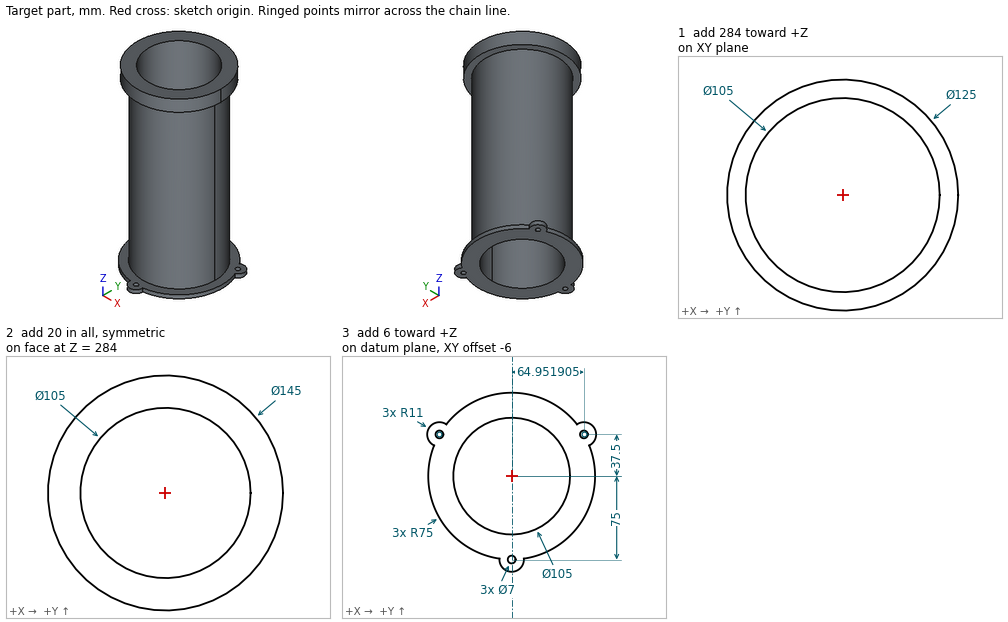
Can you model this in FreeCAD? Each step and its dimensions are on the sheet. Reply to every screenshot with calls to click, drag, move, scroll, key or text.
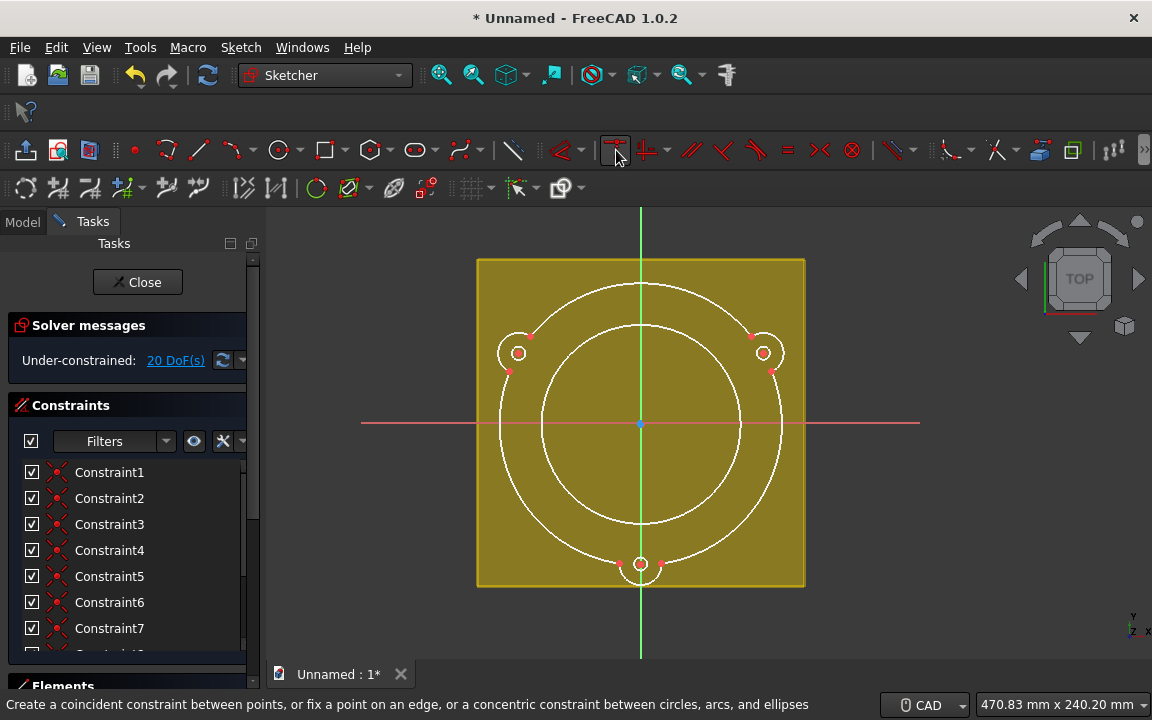
click(711, 354)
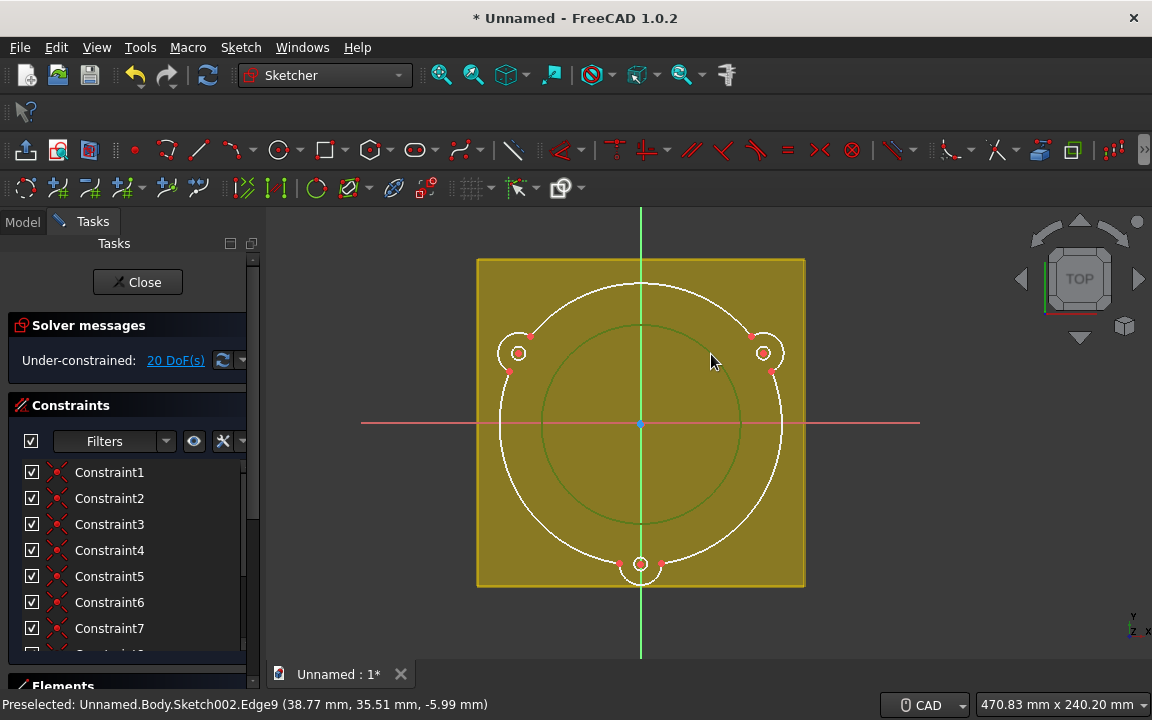
click(501, 447)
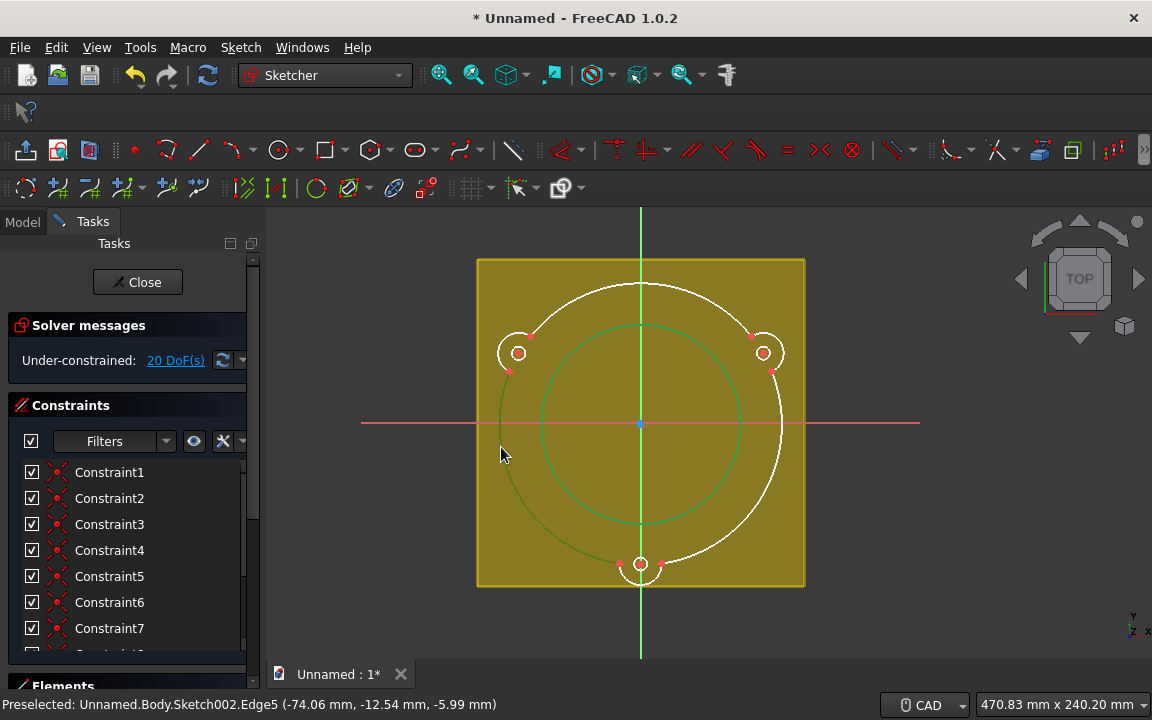
click(616, 150)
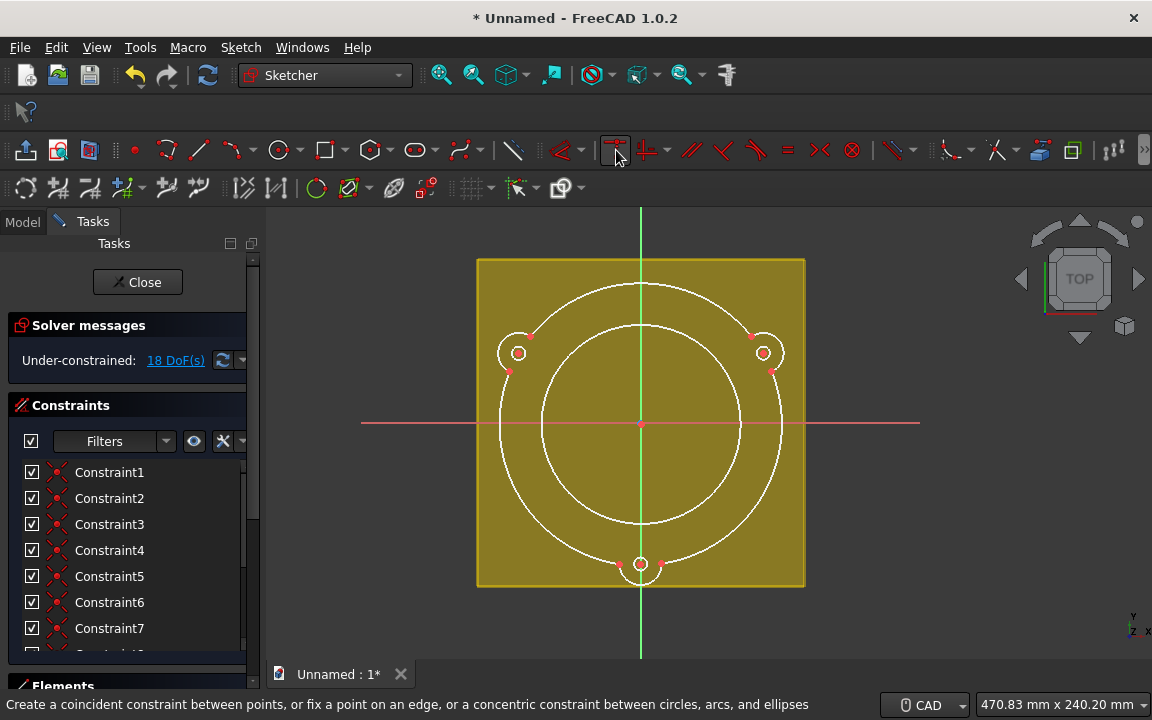
scroll(641, 424, up, 10)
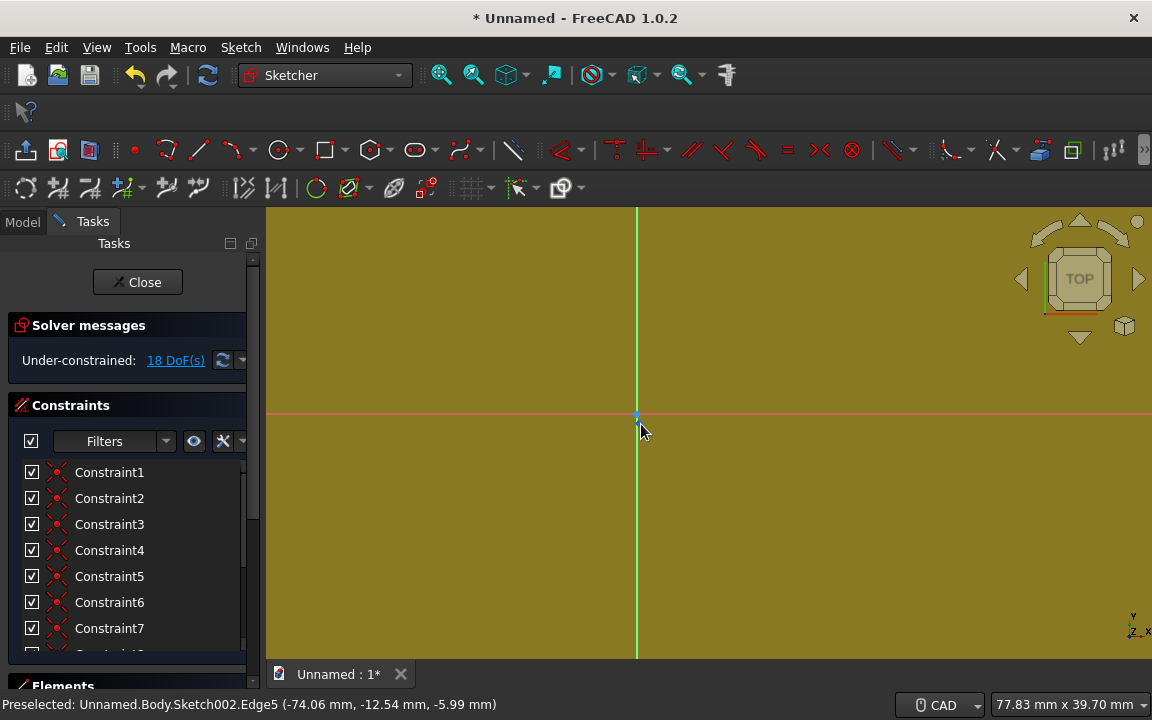
drag(627, 404, 649, 434)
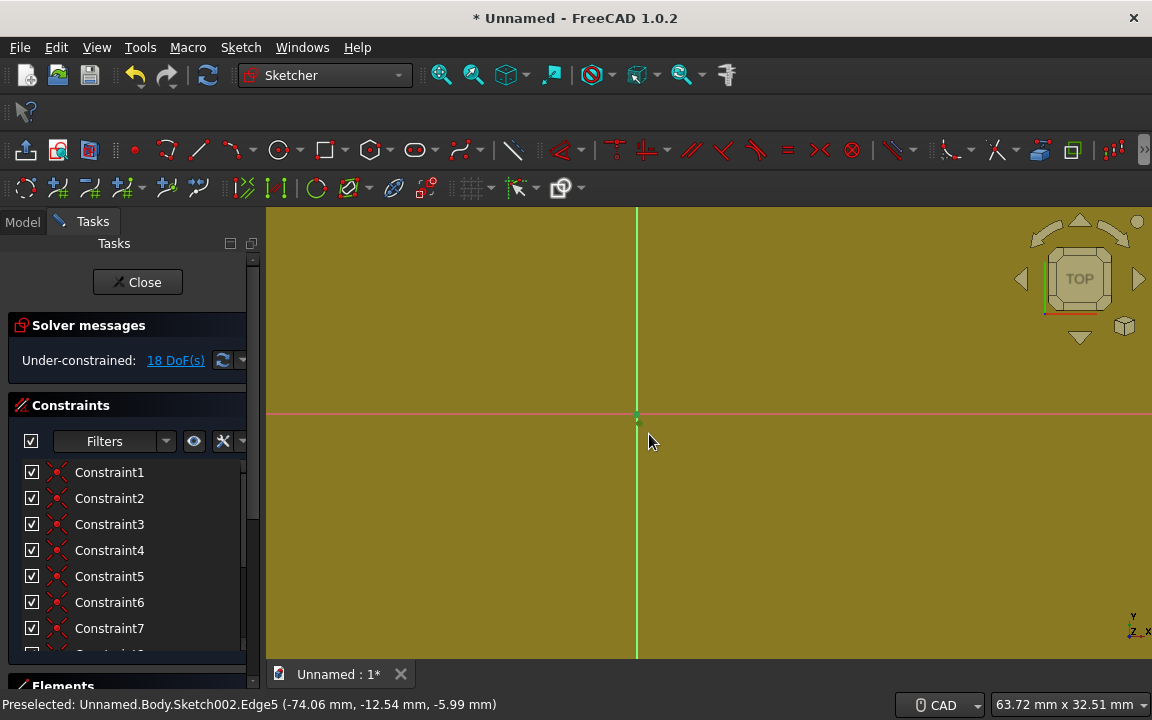
click(616, 150)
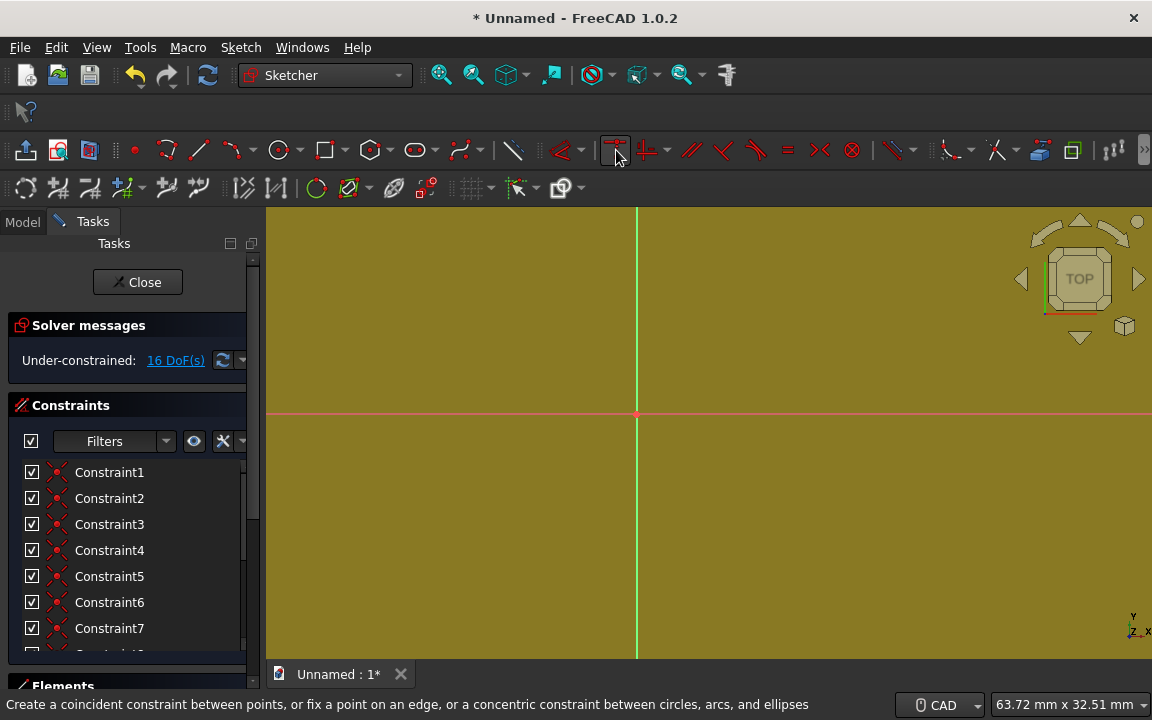
scroll(641, 424, down, 10)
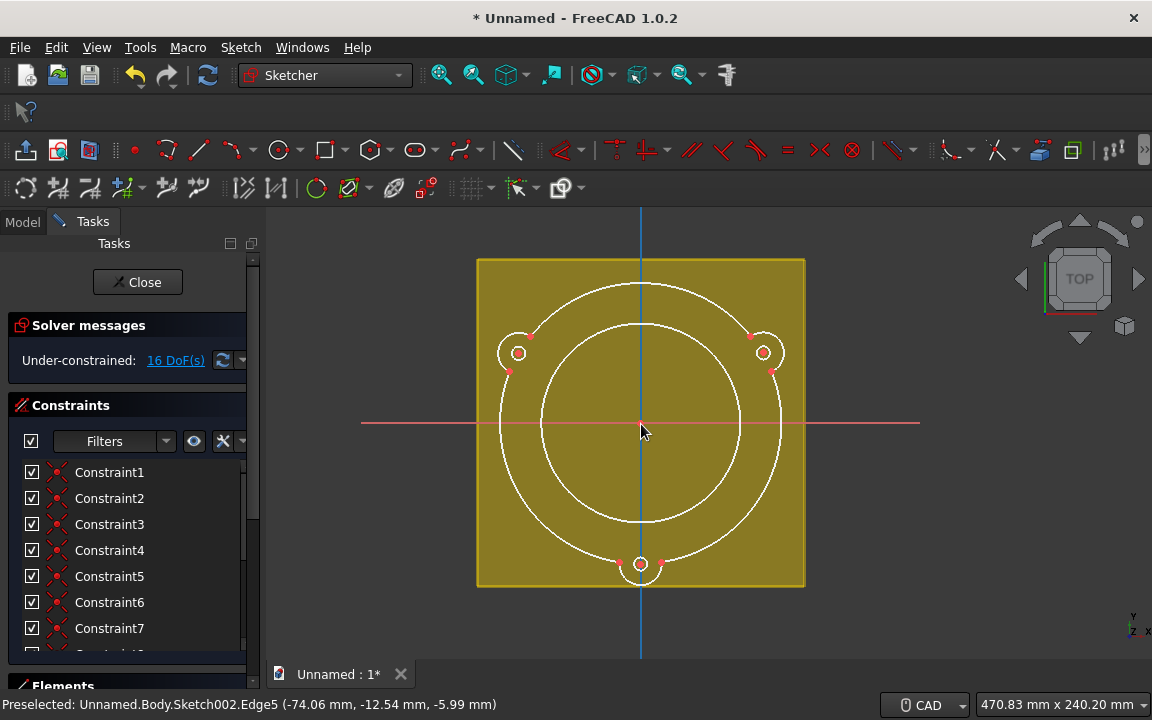
click(690, 292)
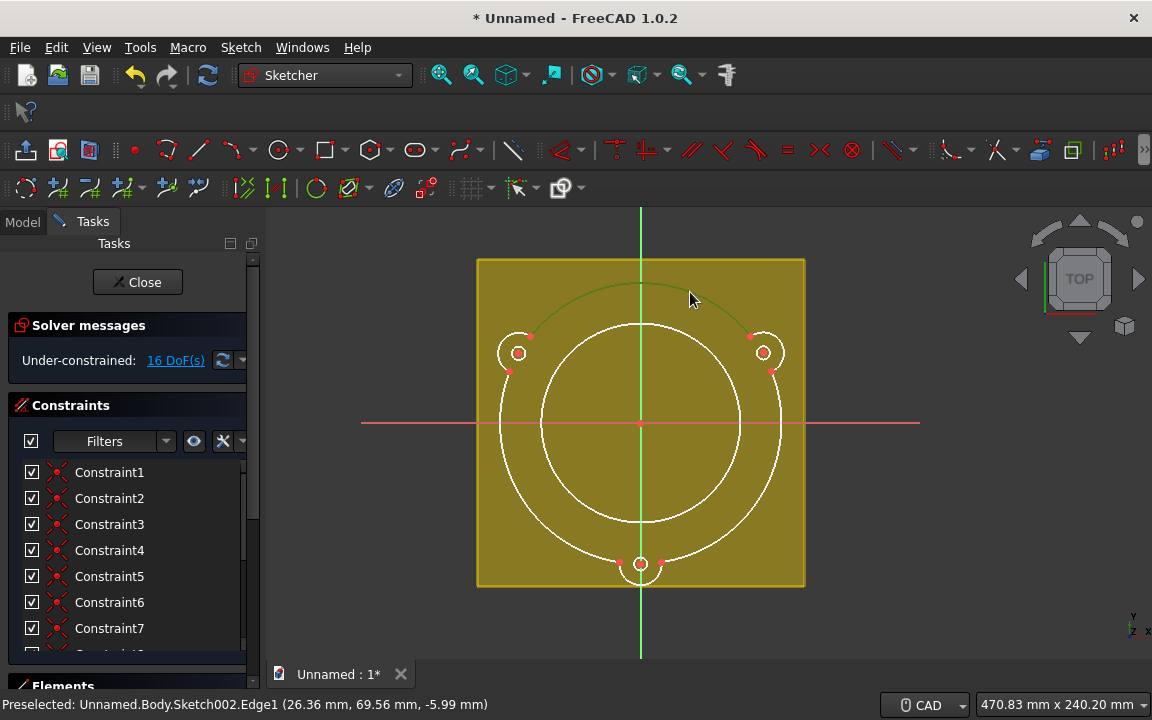
click(730, 532)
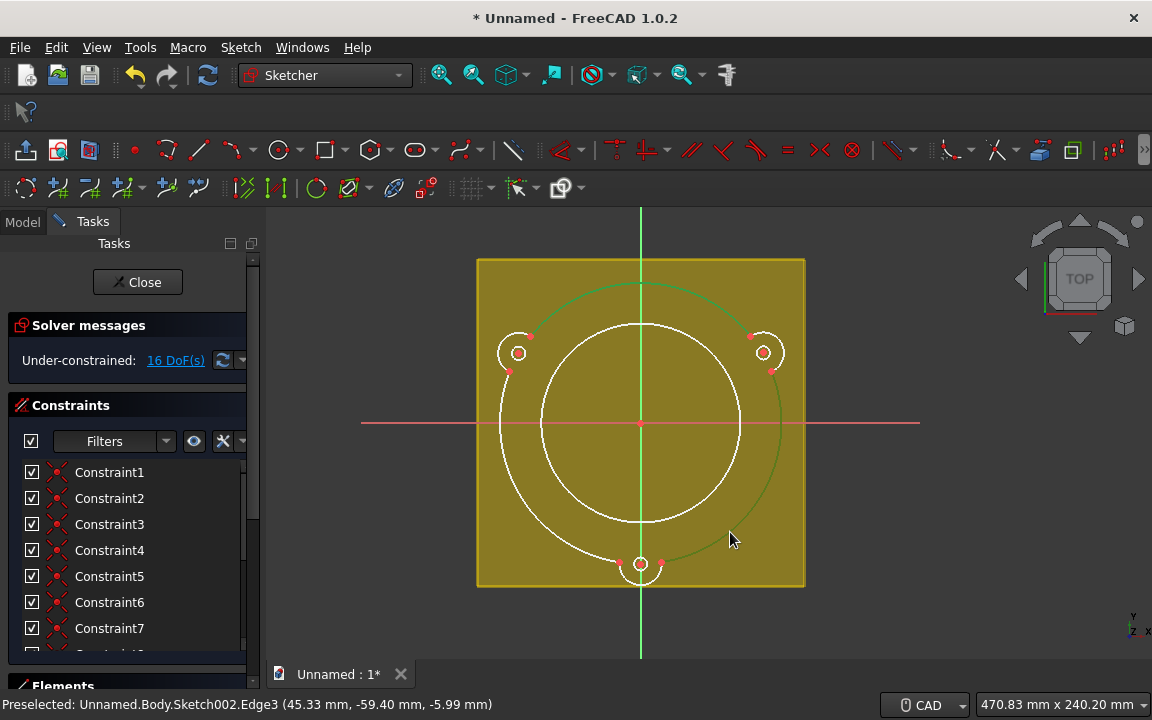
click(502, 446)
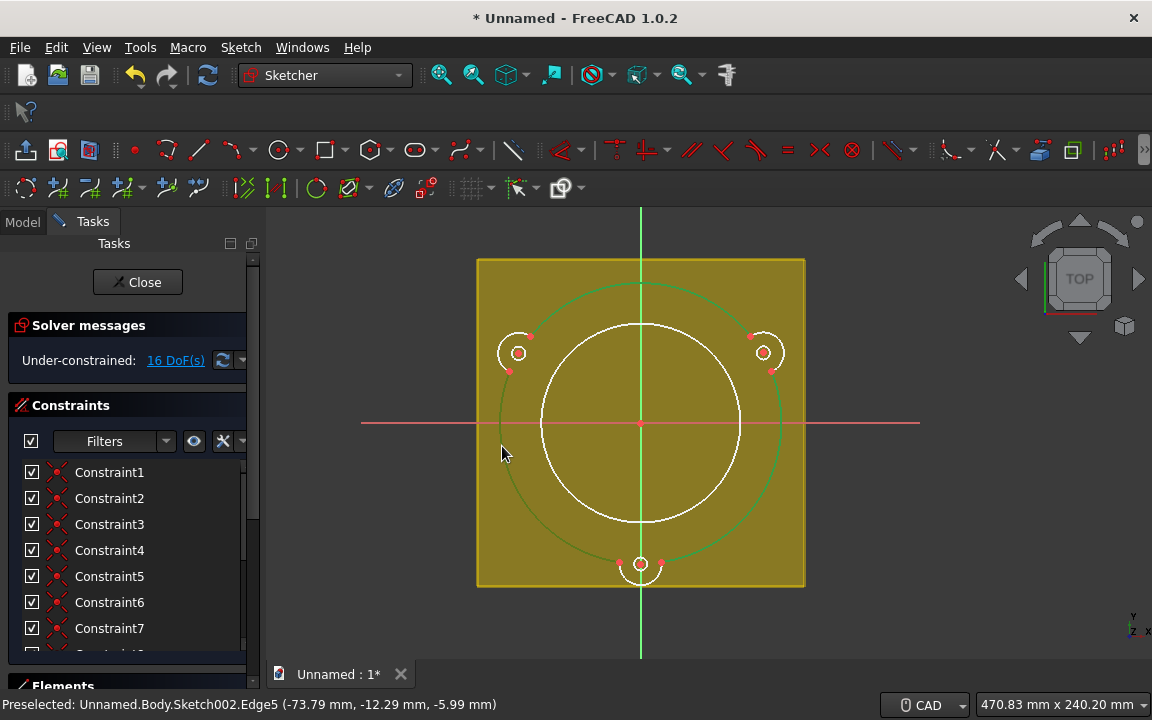
click(788, 150)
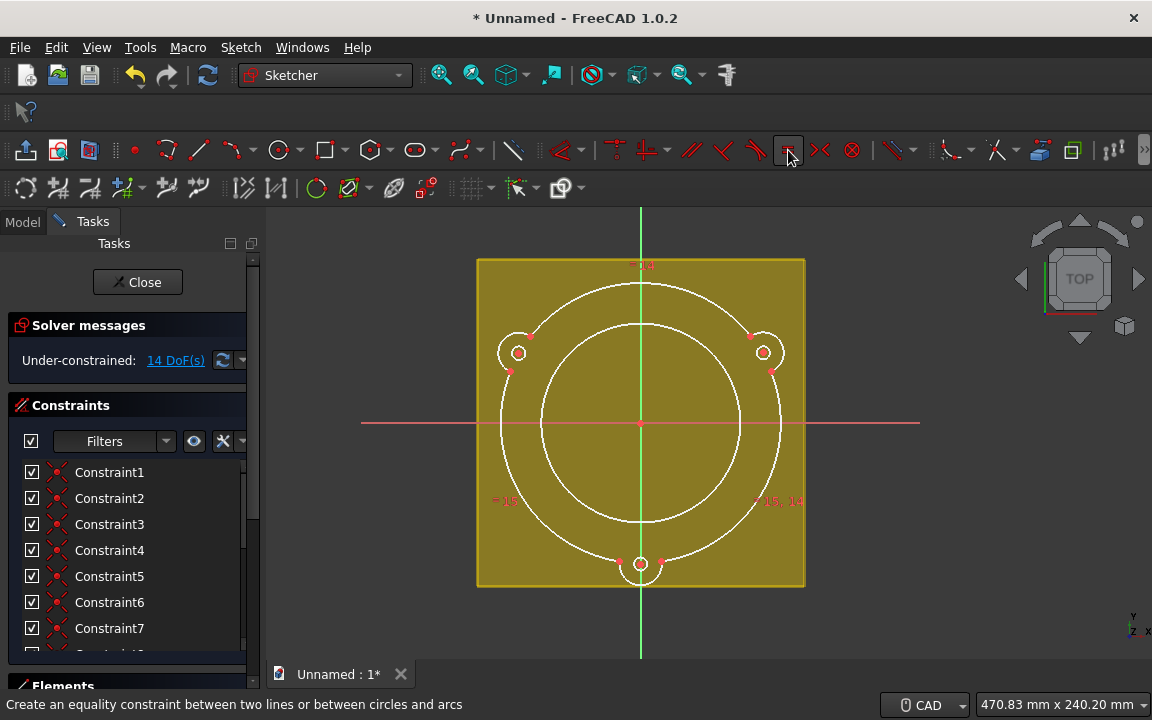
click(783, 356)